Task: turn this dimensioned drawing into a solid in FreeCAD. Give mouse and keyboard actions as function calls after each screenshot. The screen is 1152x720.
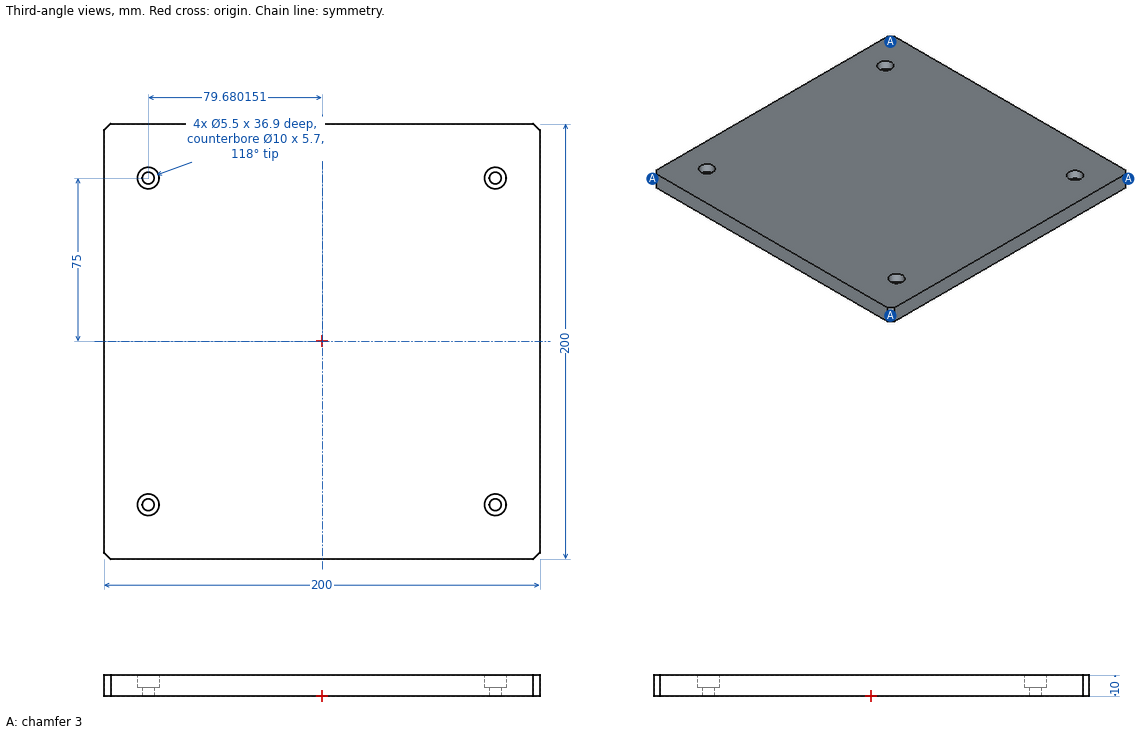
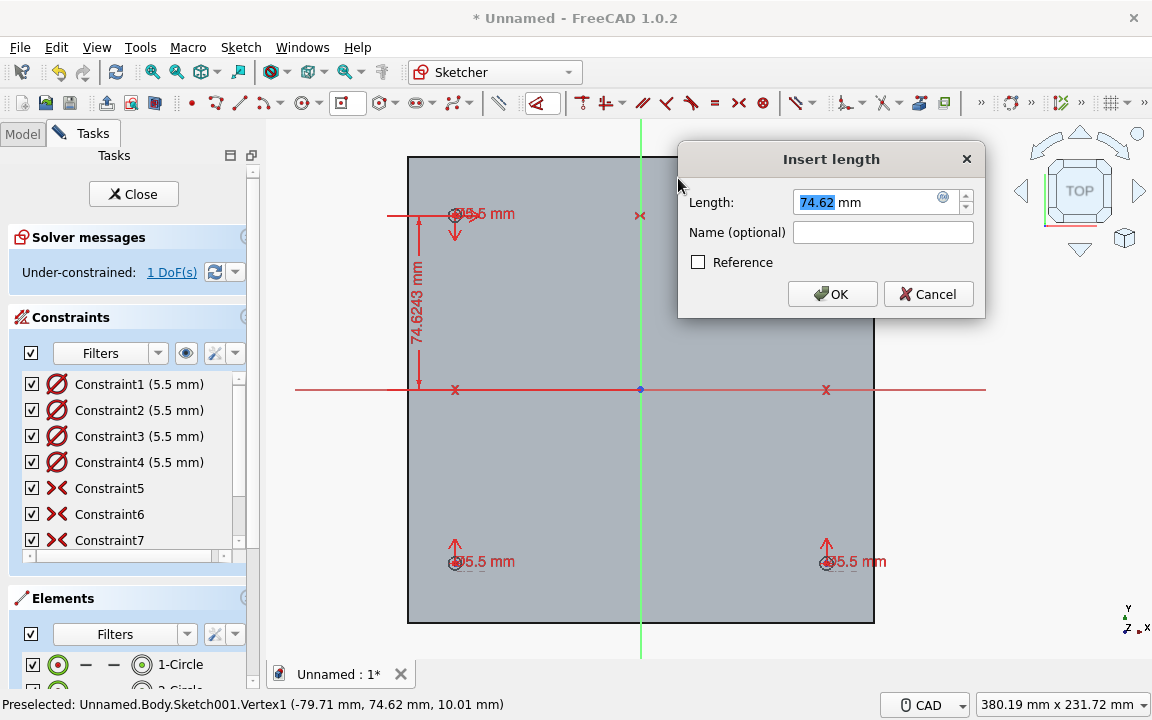
text(75)
key(Return)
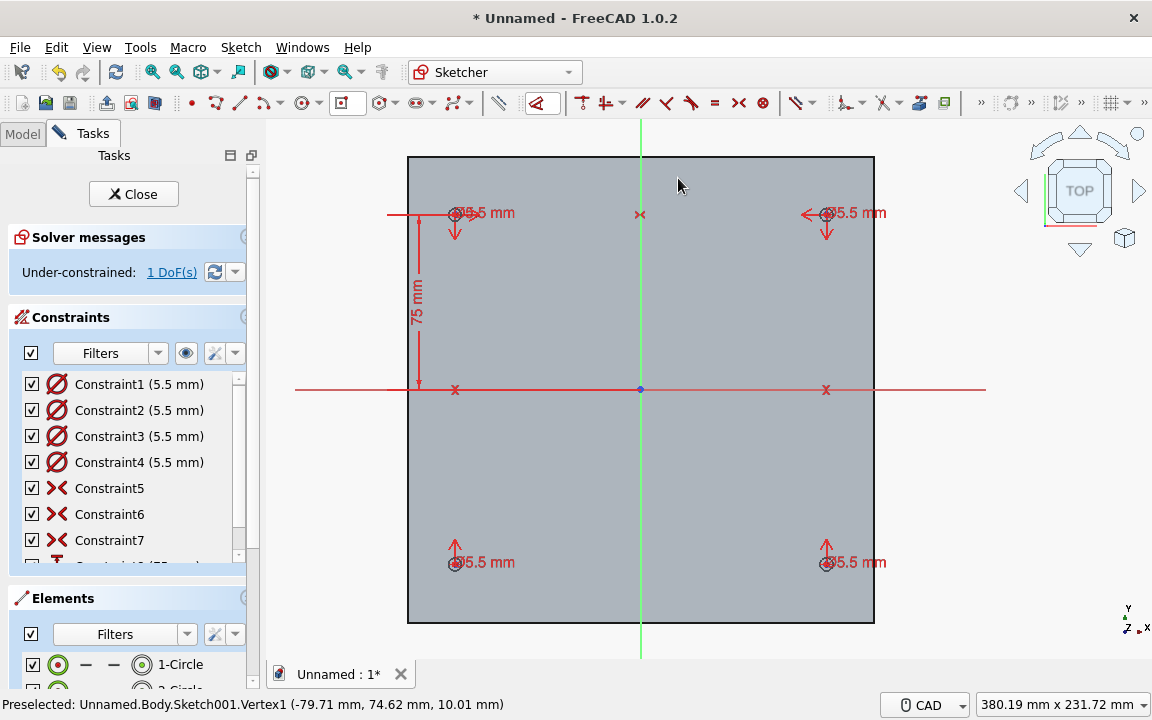
click(455, 215)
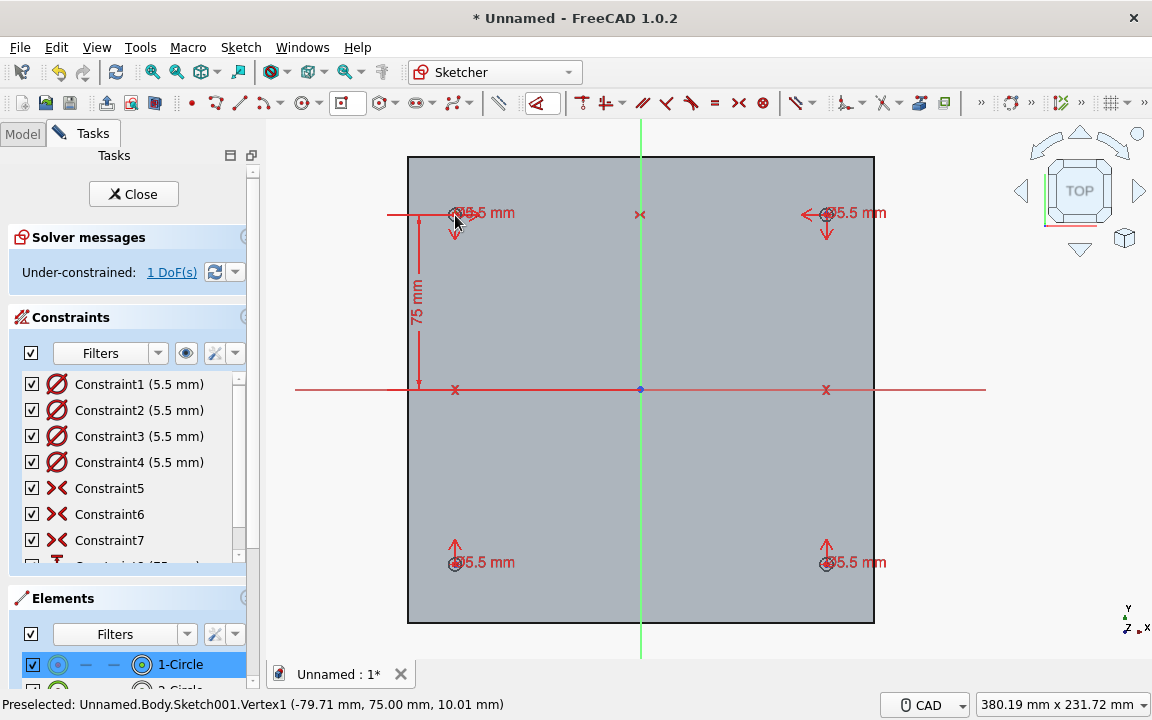
key(l)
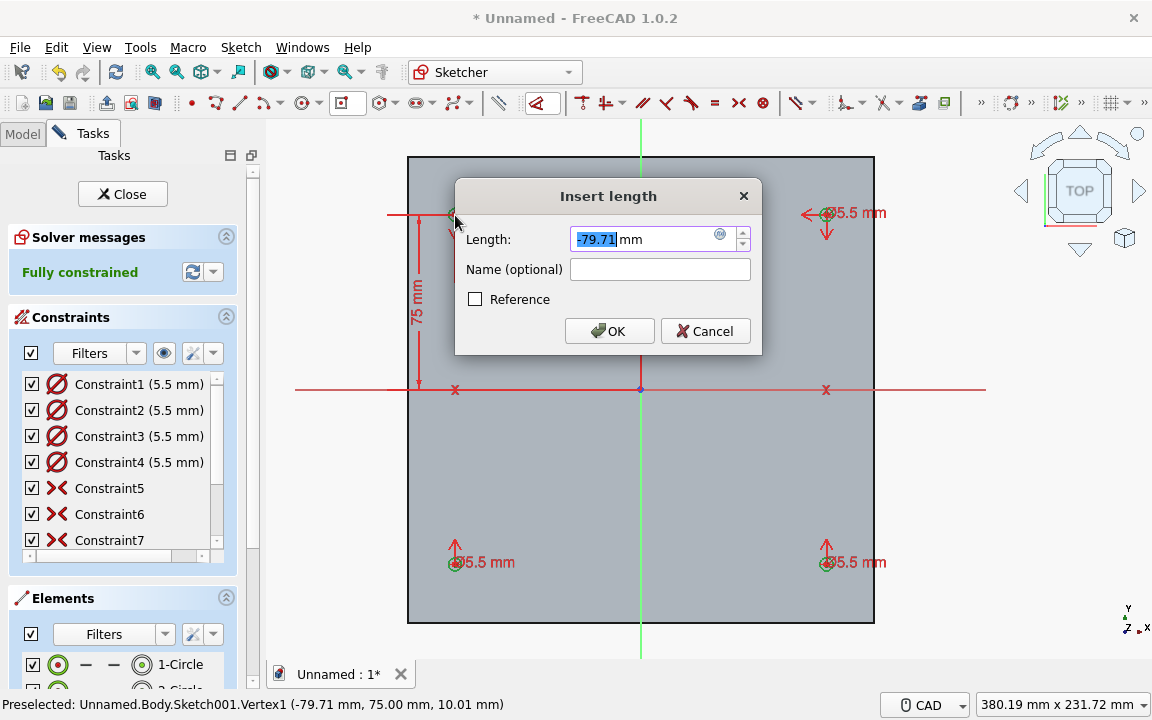
text(-79.680151)
key(Return)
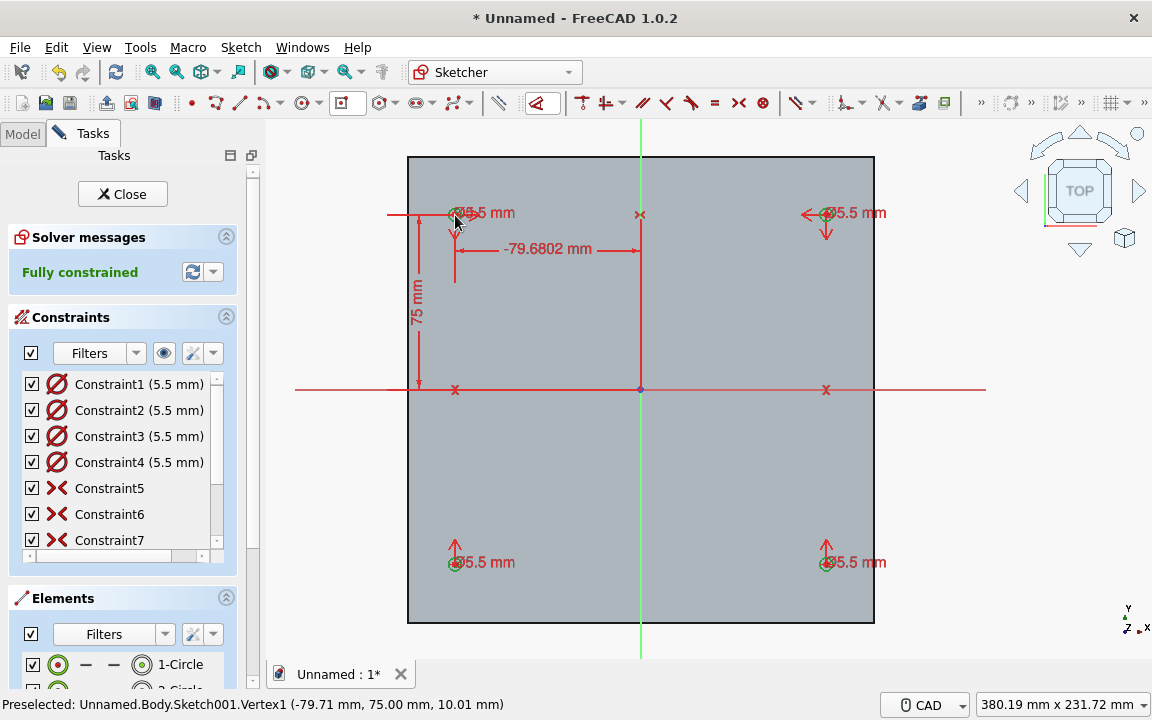
click(123, 194)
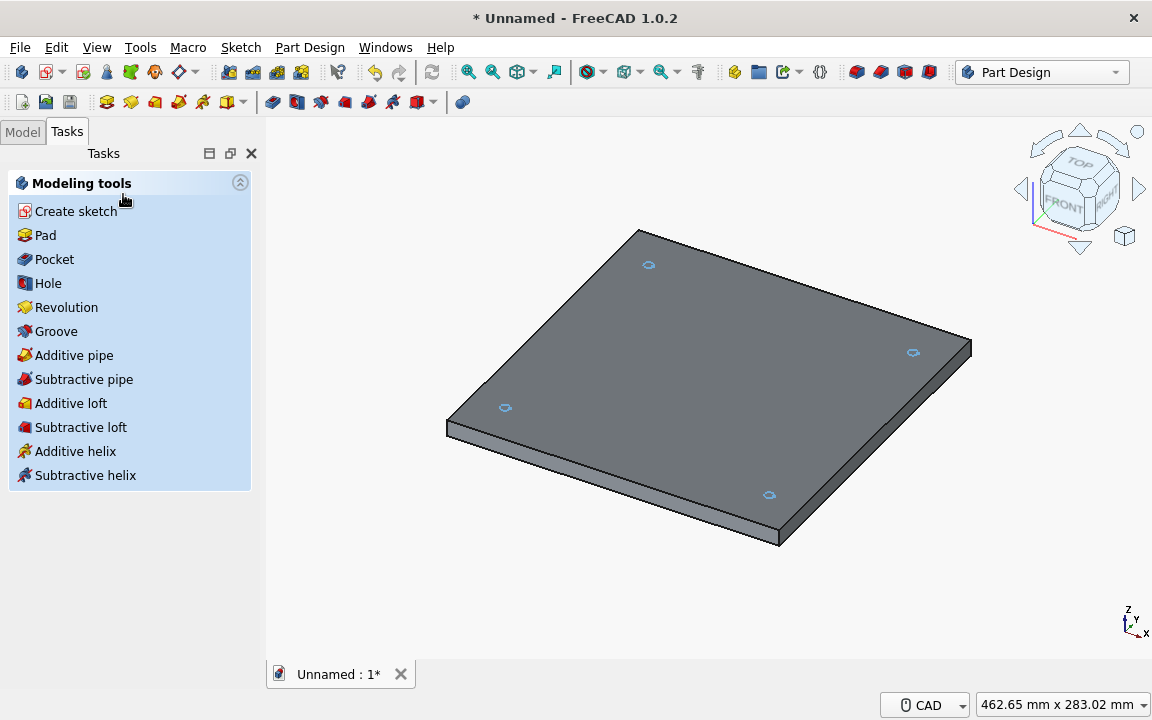
click(298, 102)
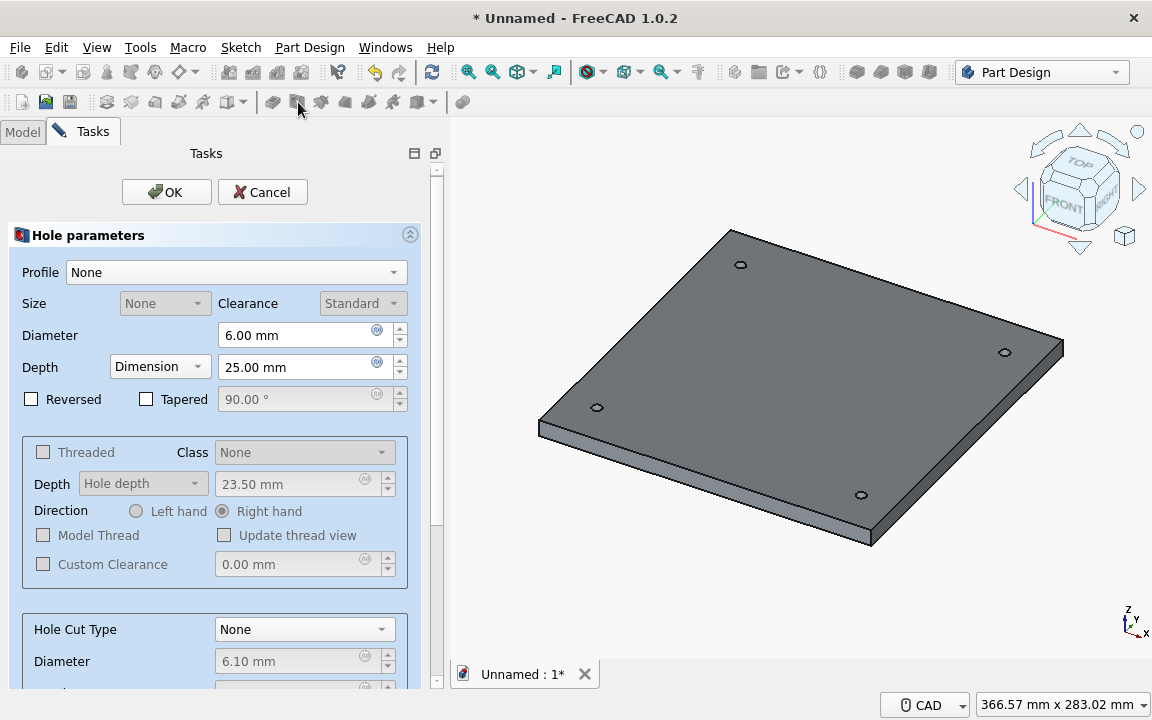
triple_click(305, 335)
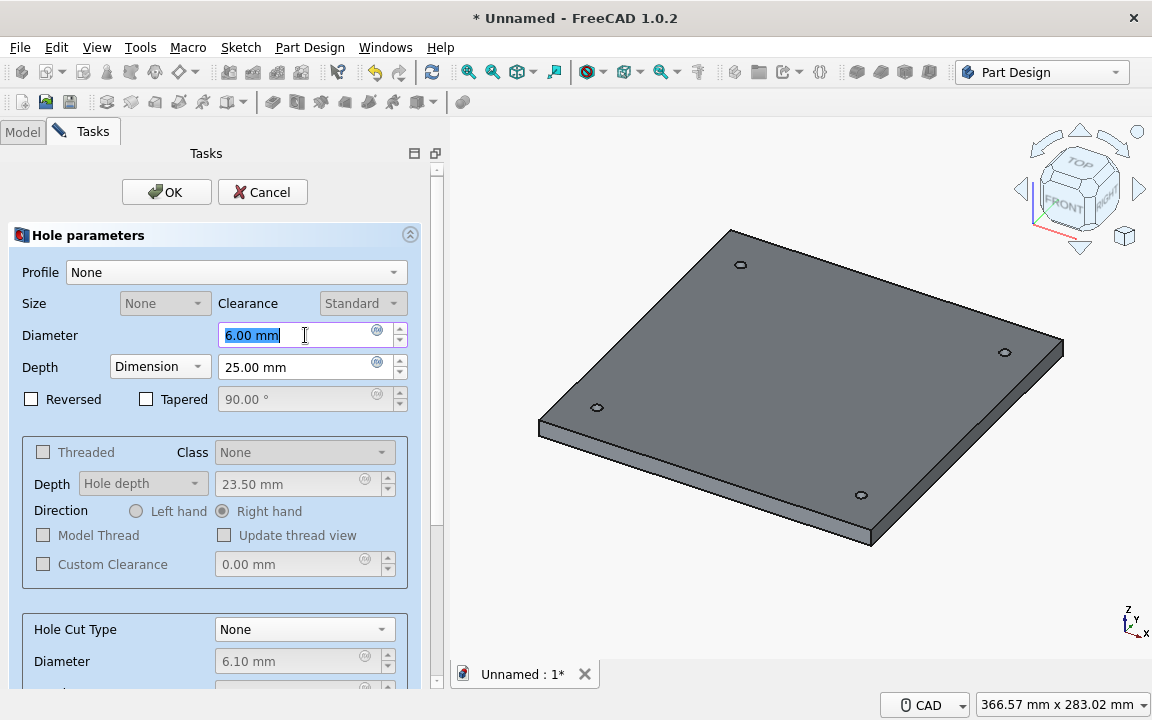
text(5.5)
key(Tab)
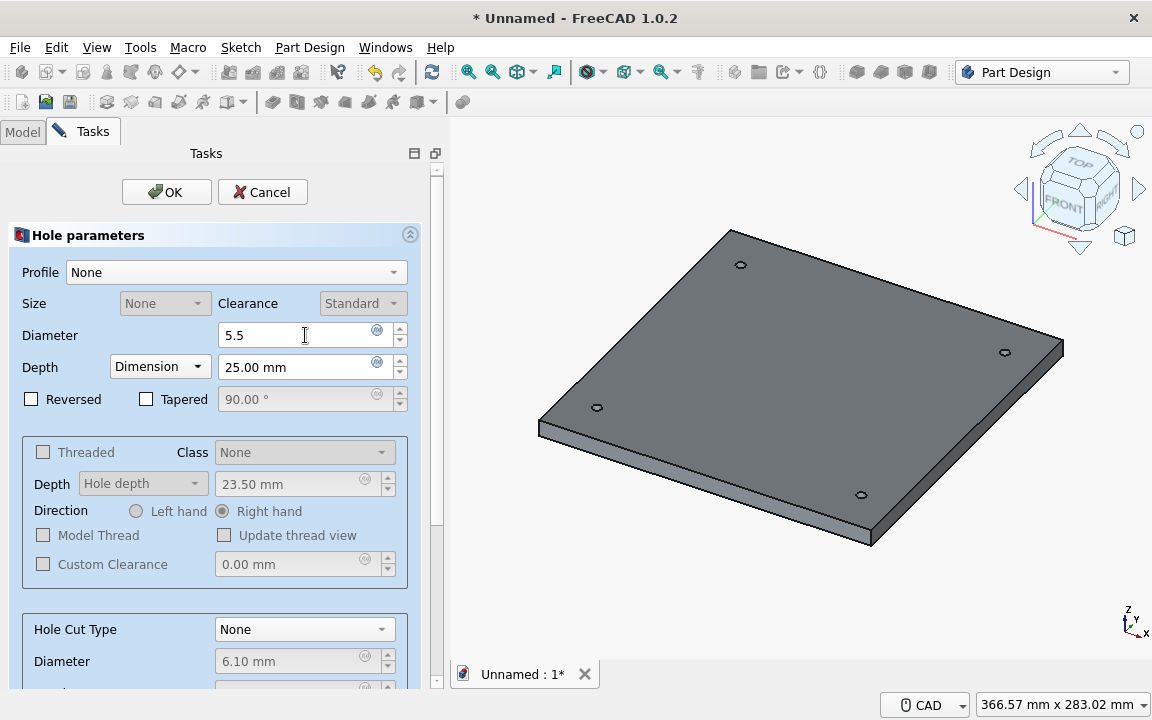
triple_click(305, 367)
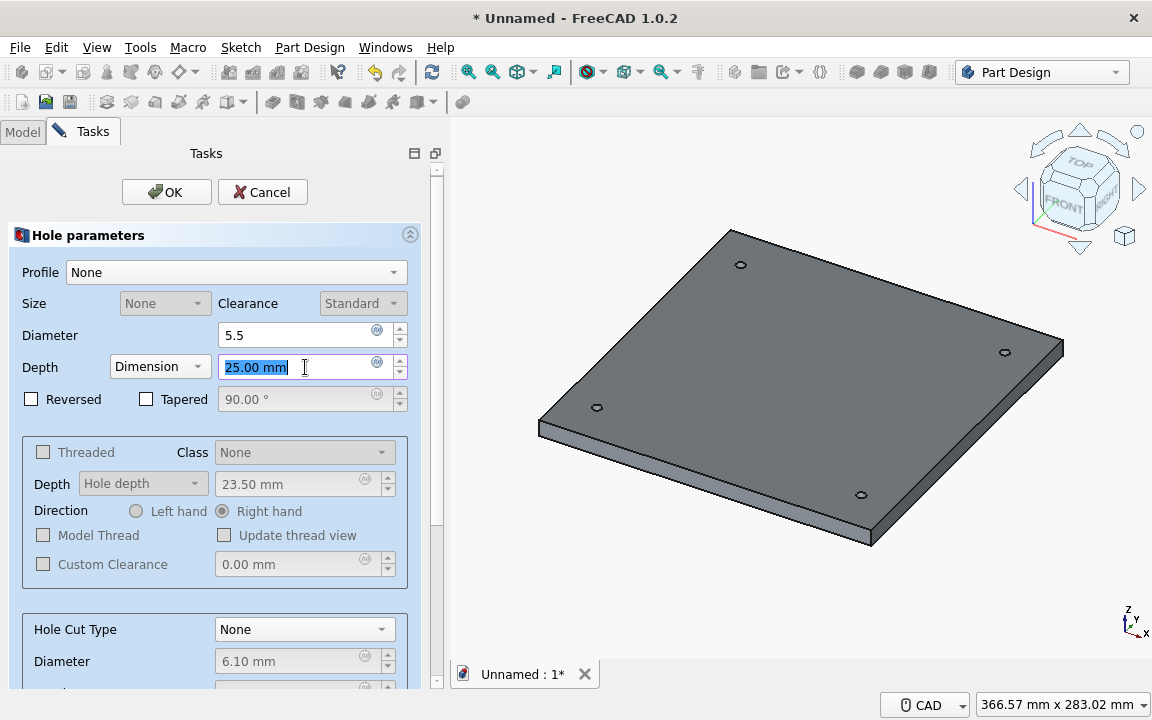
text(36.9)
key(Tab)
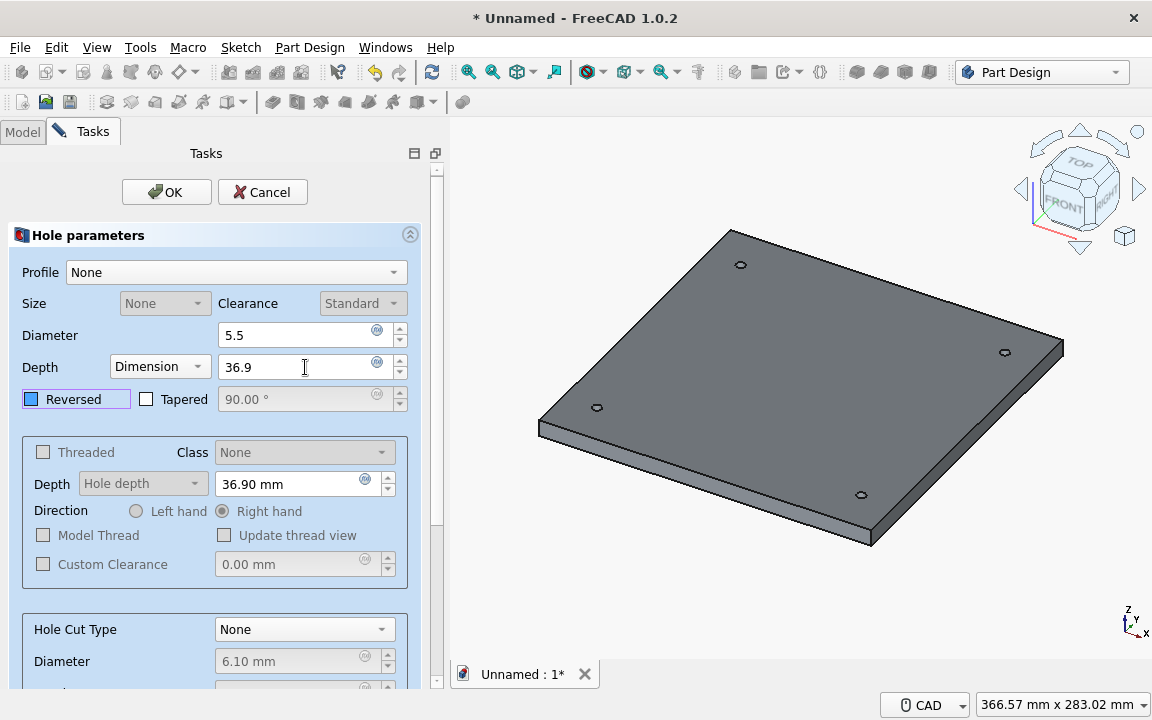
click(306, 630)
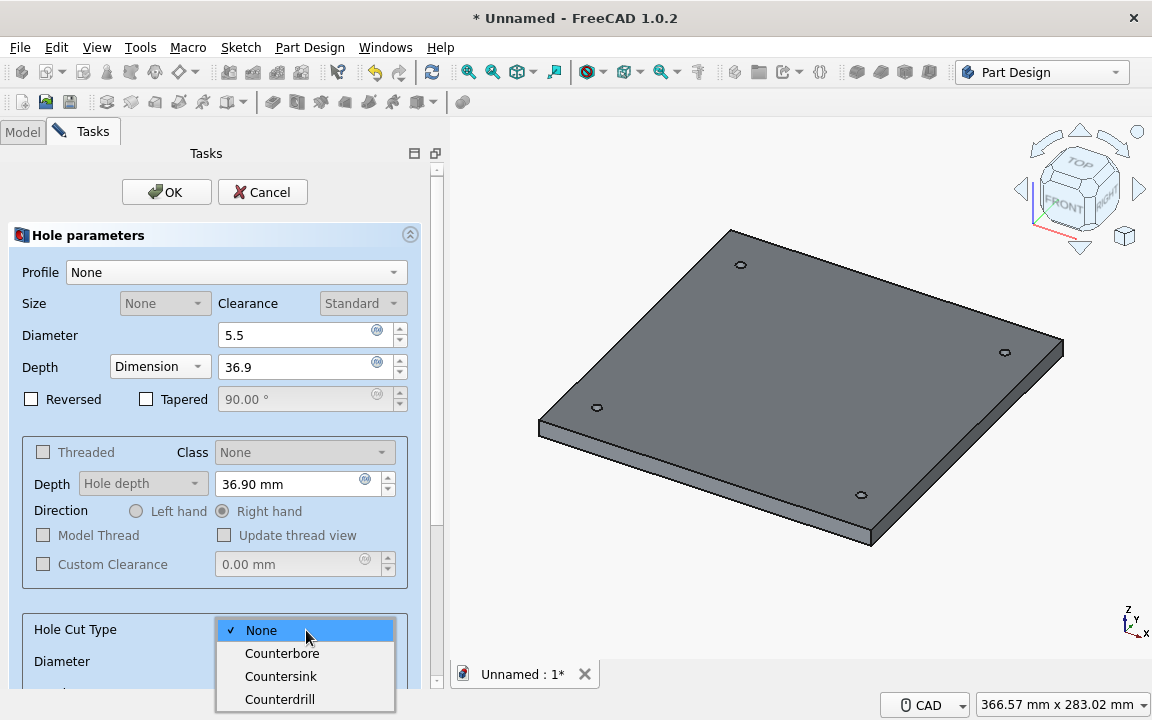
click(304, 654)